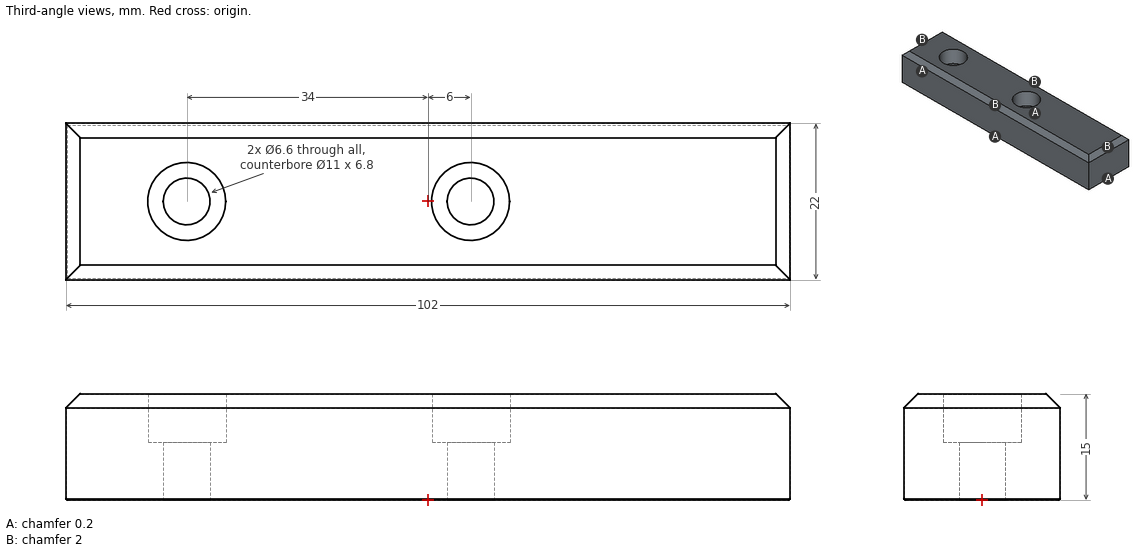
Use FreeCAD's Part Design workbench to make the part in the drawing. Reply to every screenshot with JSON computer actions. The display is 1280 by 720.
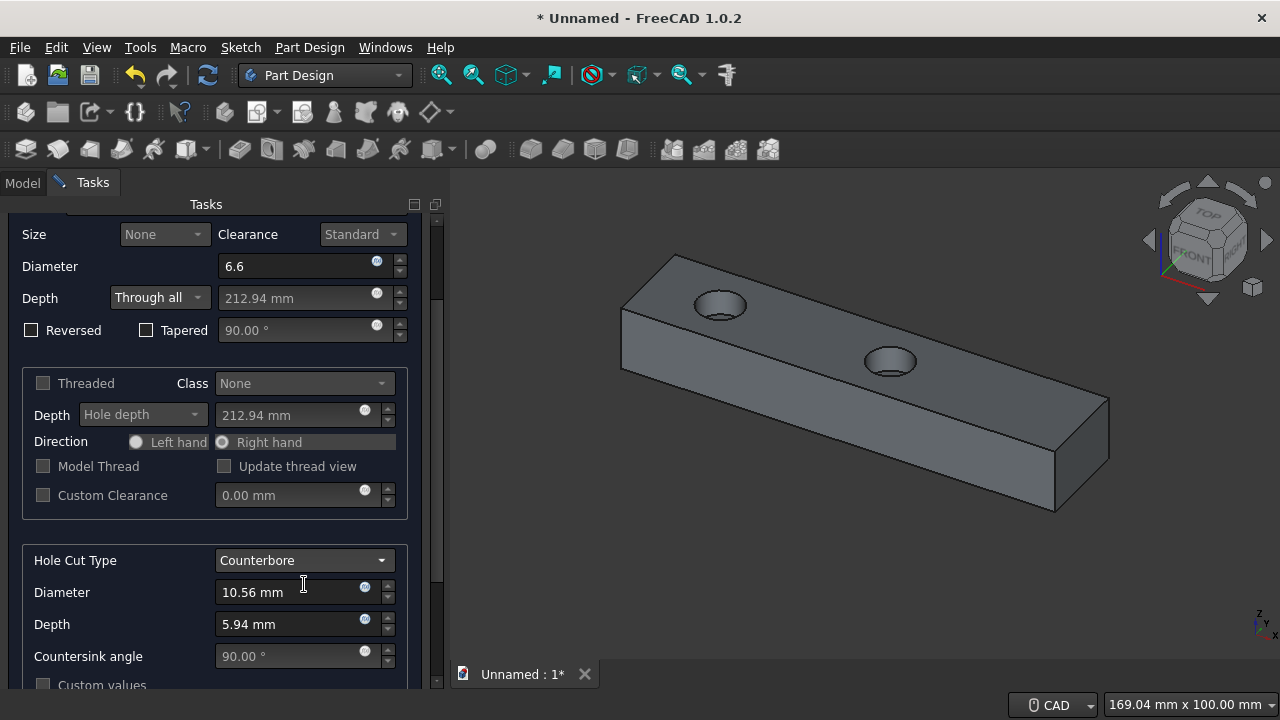
{"action": "triple_click", "coordinate": [298, 592]}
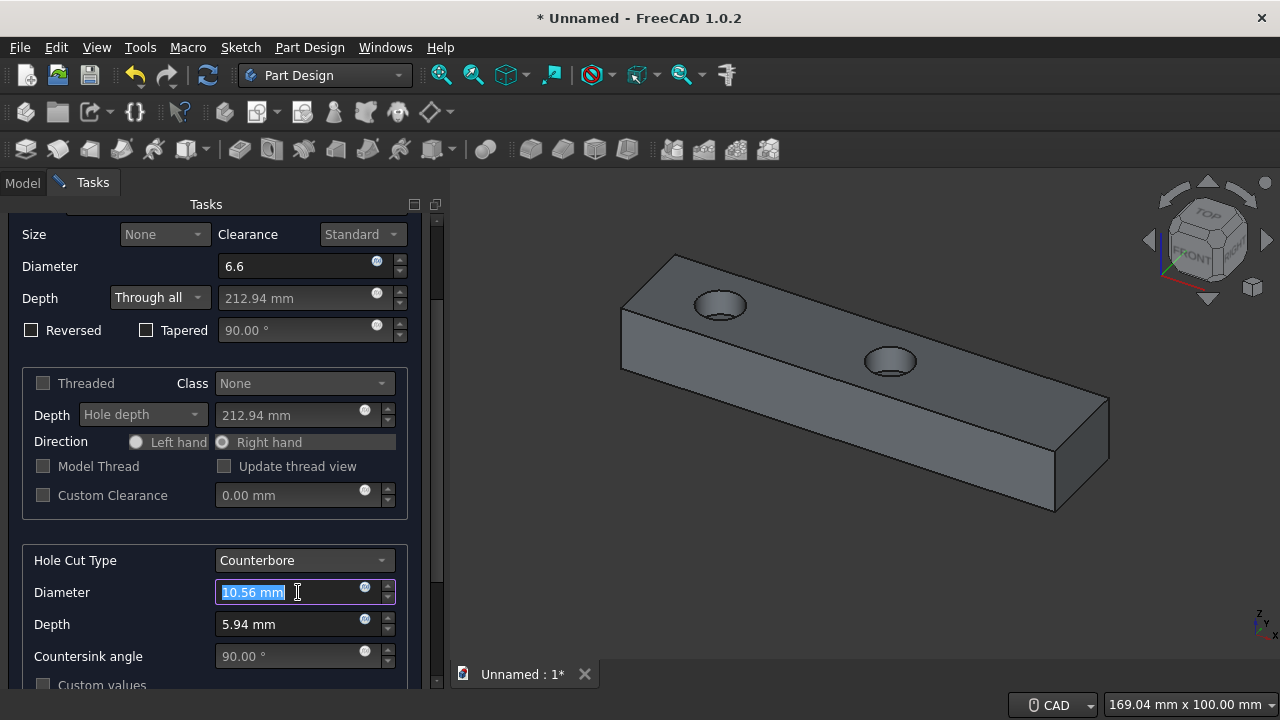
{"action": "type", "text": "11"}
{"action": "key", "text": "Tab"}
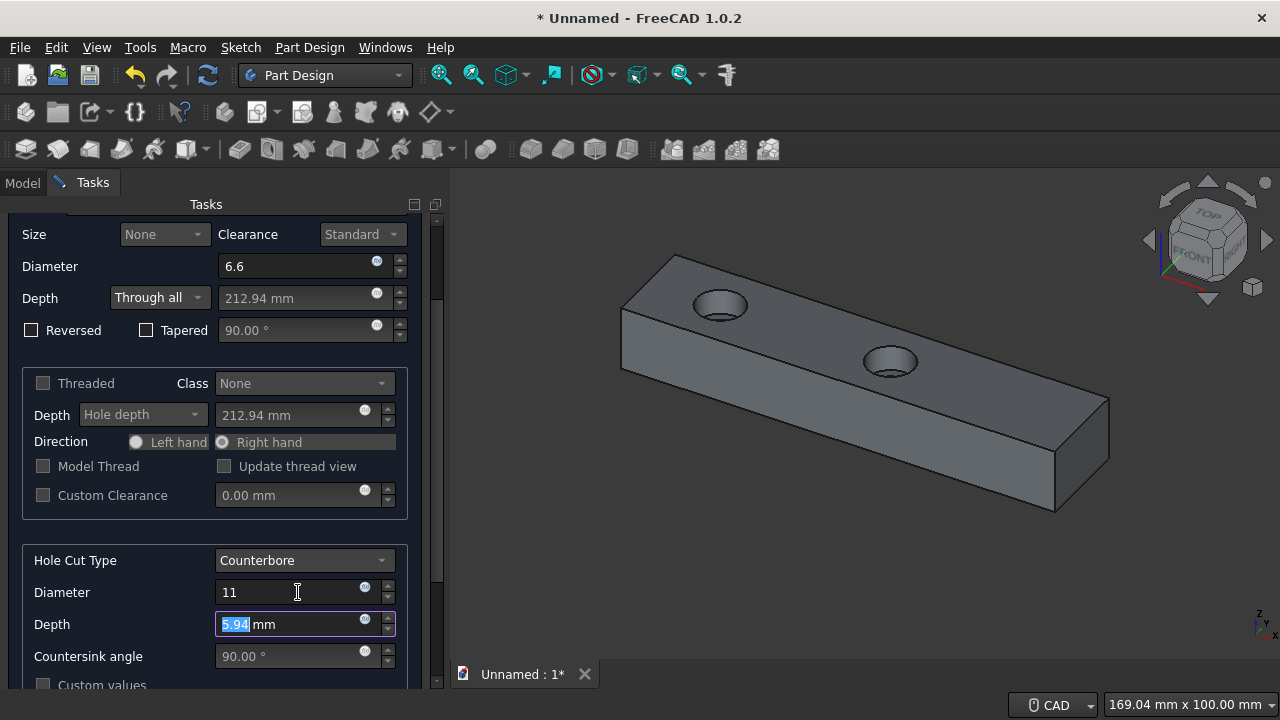
{"action": "type", "text": "6.8"}
{"action": "key", "text": "Tab"}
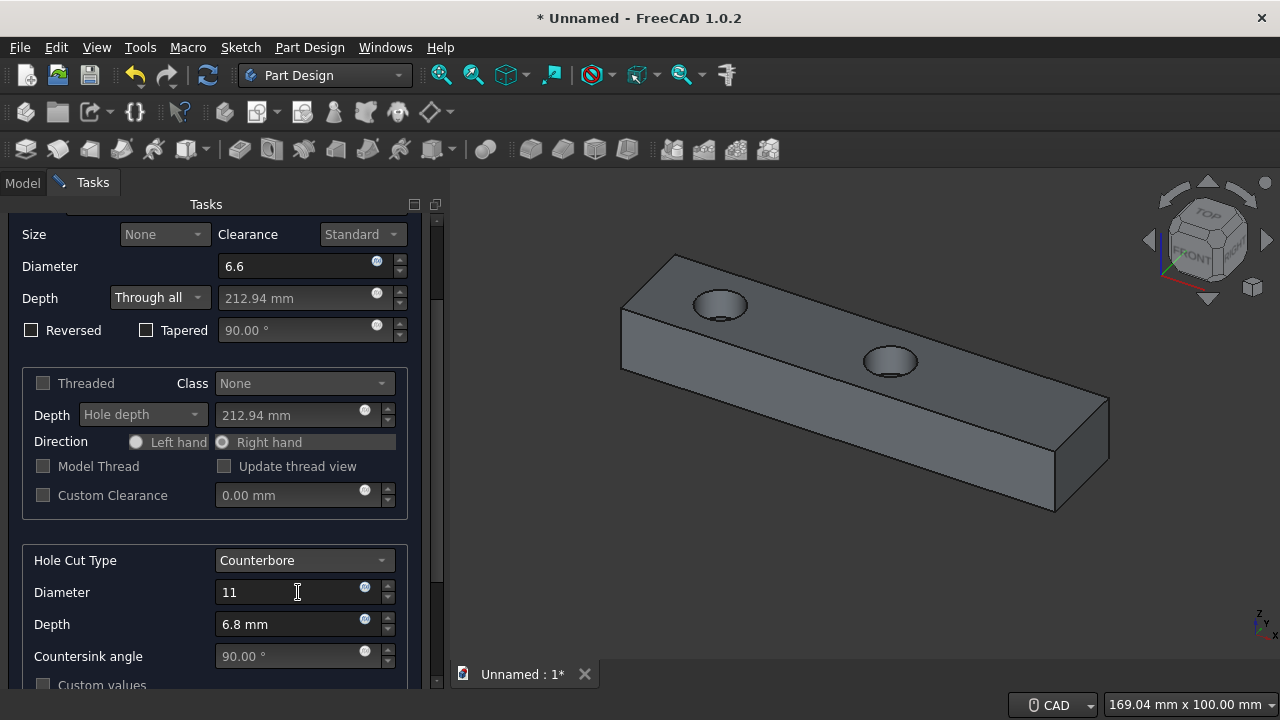
{"action": "scroll", "coordinate": [437, 451], "scroll_direction": "up", "scroll_amount": 3}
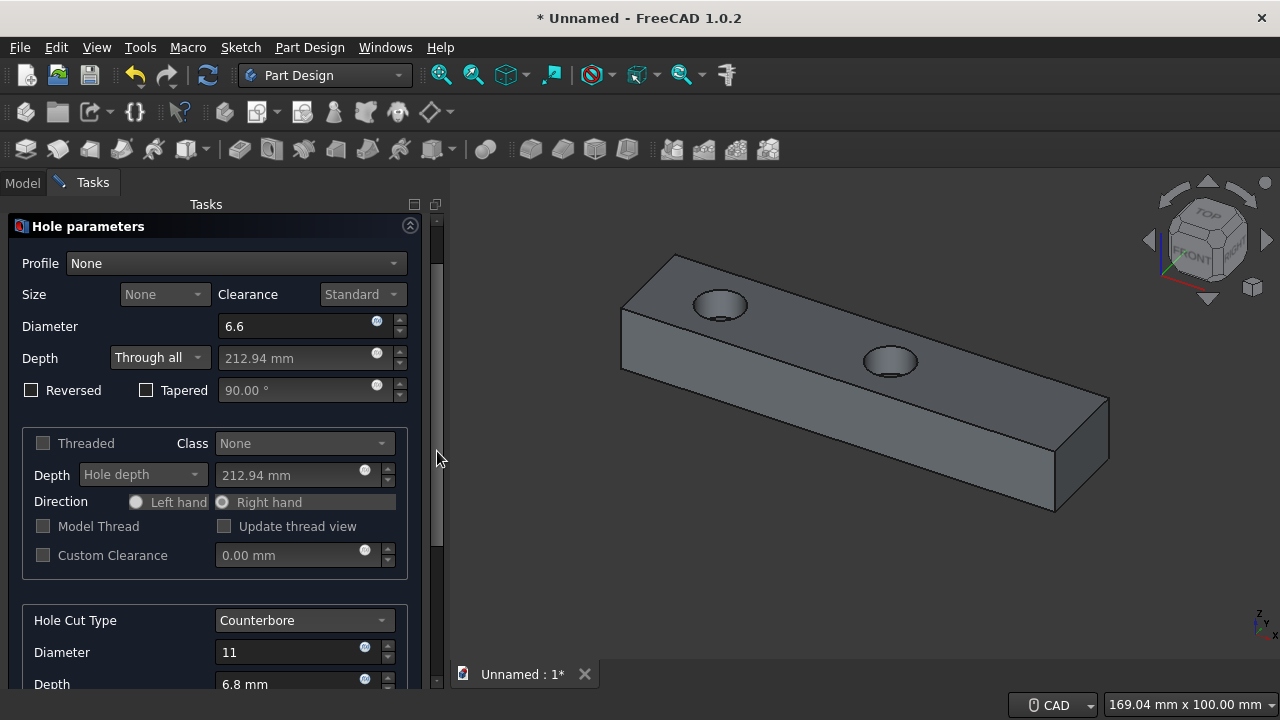
{"action": "left_click", "coordinate": [167, 243]}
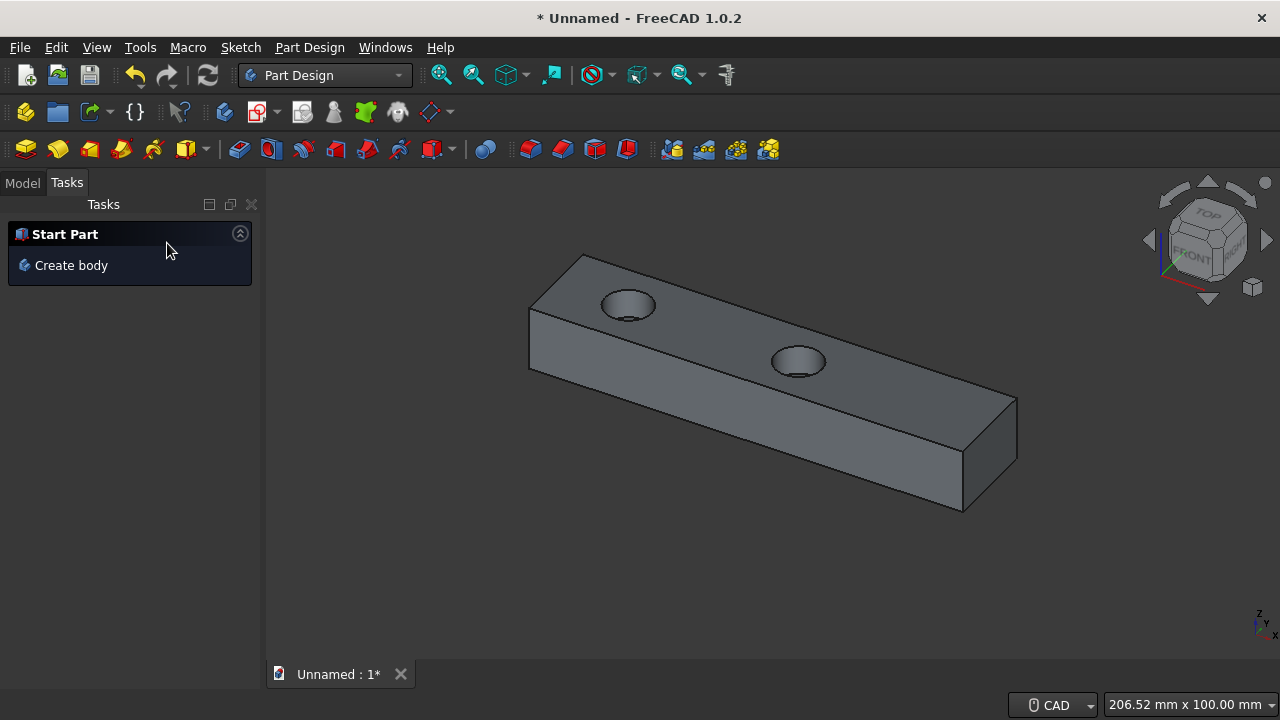
{"action": "key", "text": "0"}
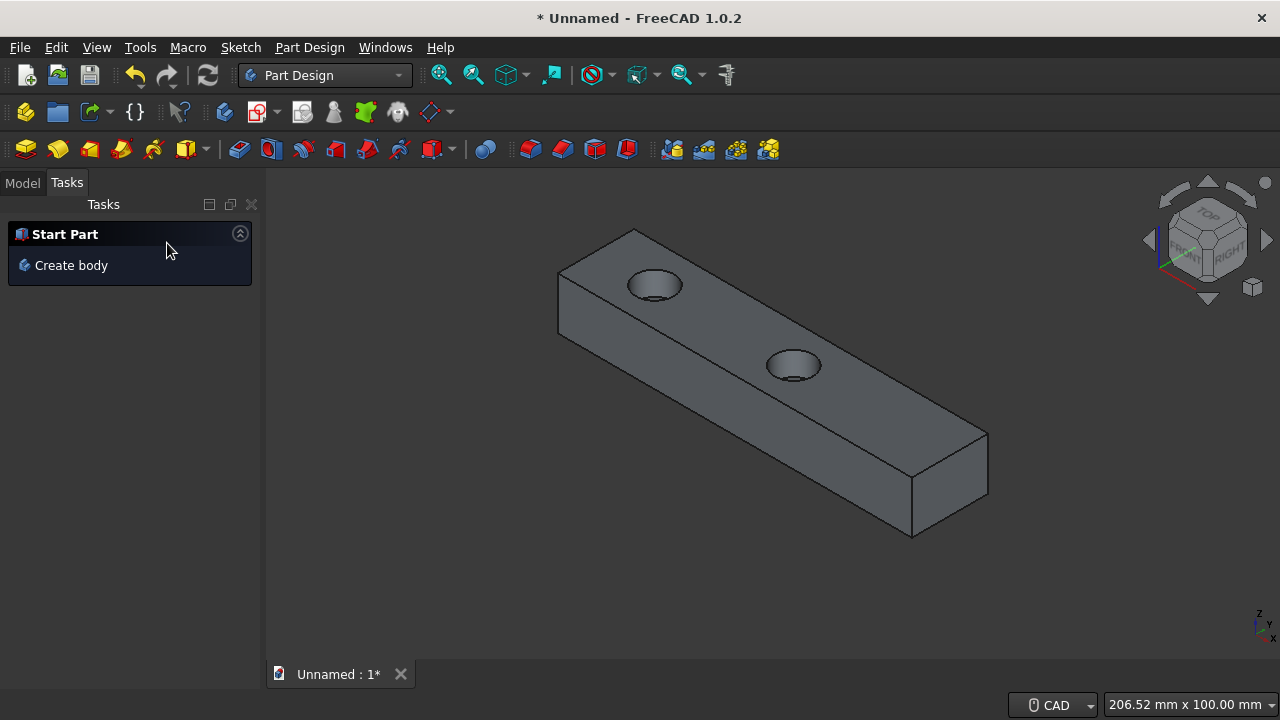
{"action": "key", "text": "2"}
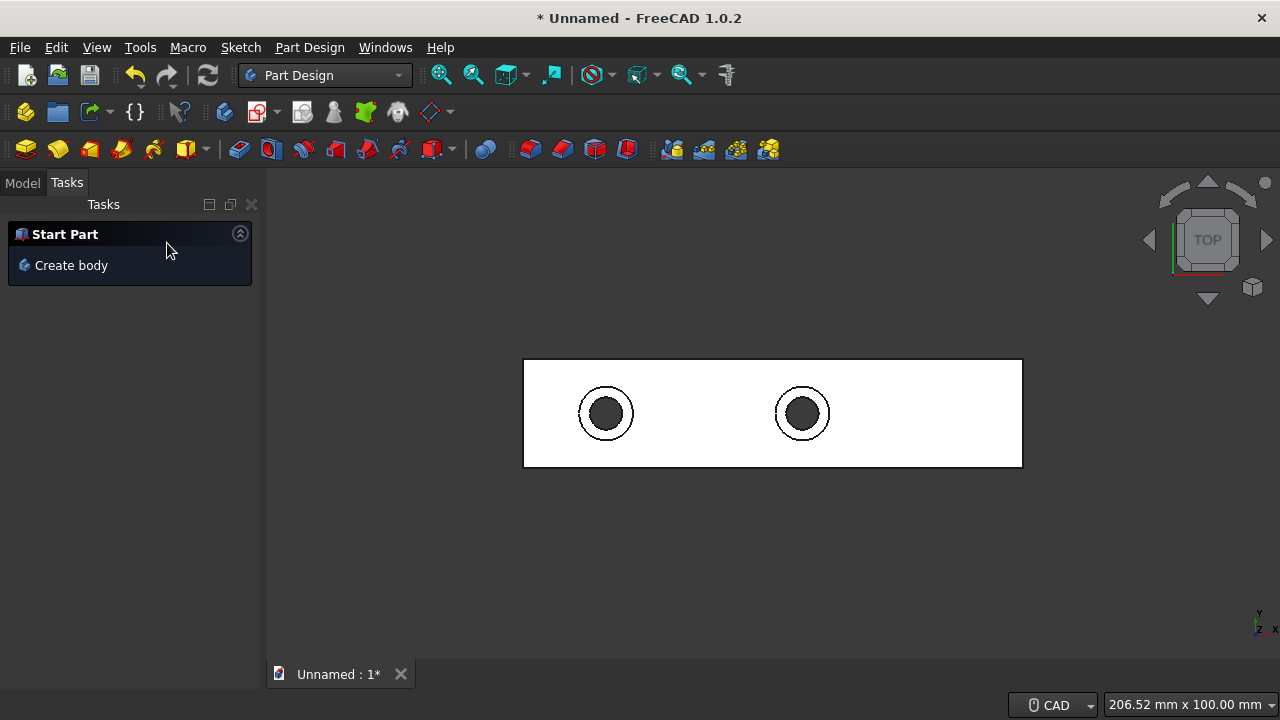
{"action": "key", "text": "1"}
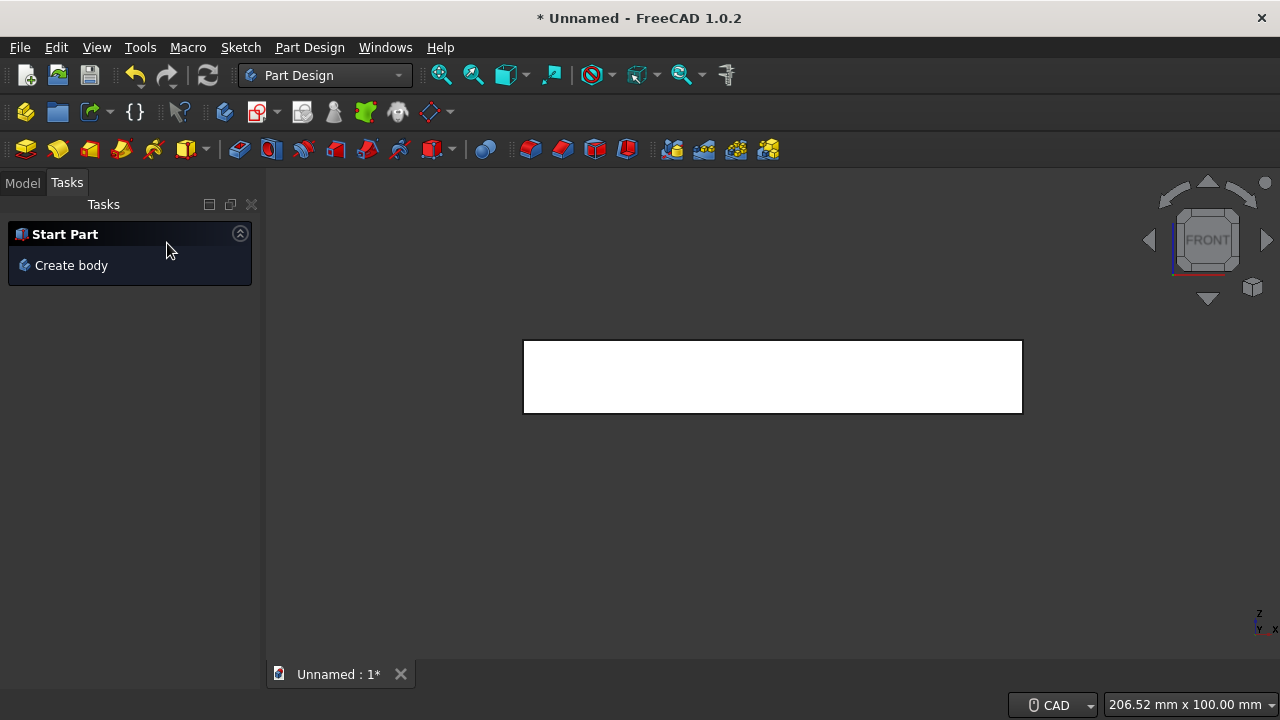
{"action": "left_click", "coordinate": [773, 412]}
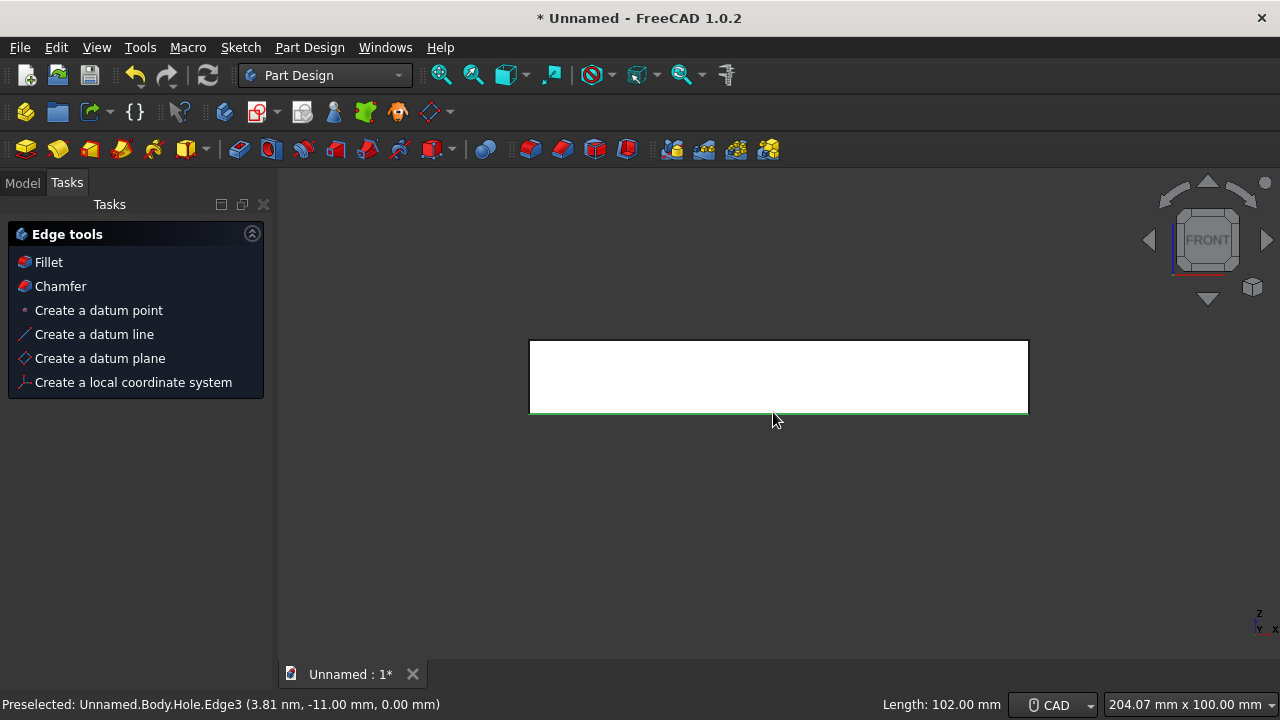
{"action": "key", "text": "3"}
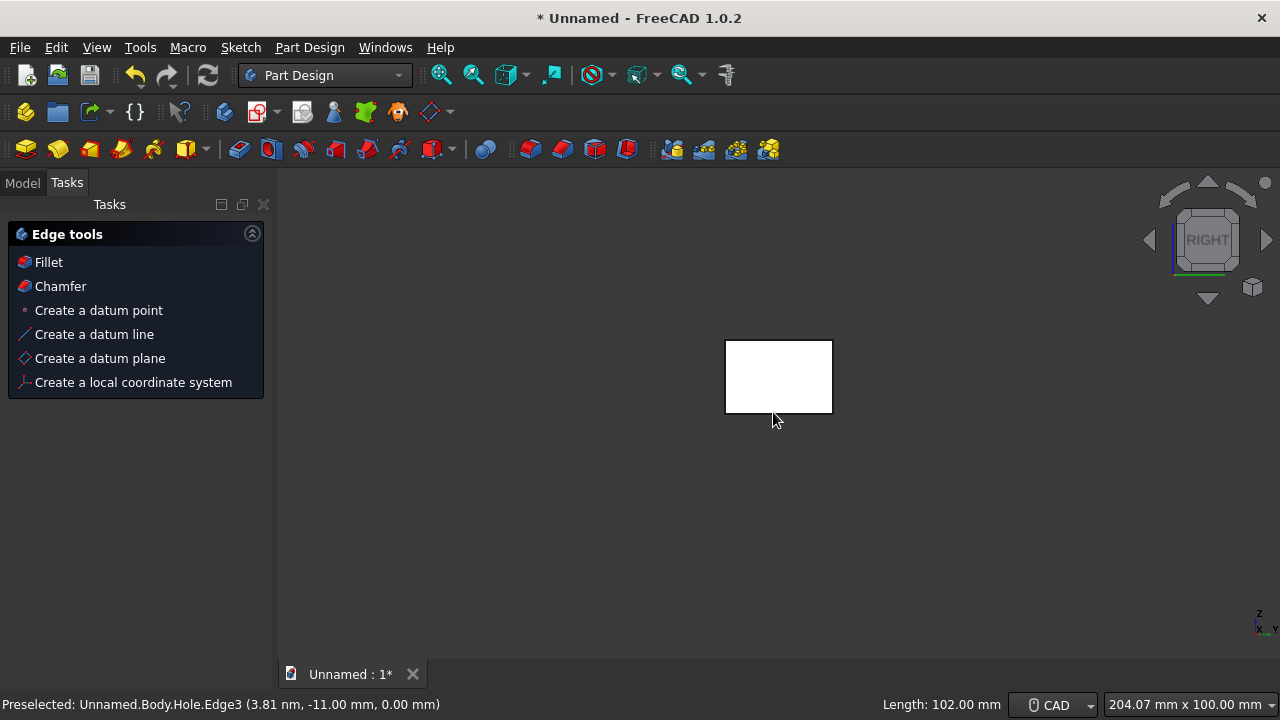
{"action": "left_click", "coordinate": [442, 76]}